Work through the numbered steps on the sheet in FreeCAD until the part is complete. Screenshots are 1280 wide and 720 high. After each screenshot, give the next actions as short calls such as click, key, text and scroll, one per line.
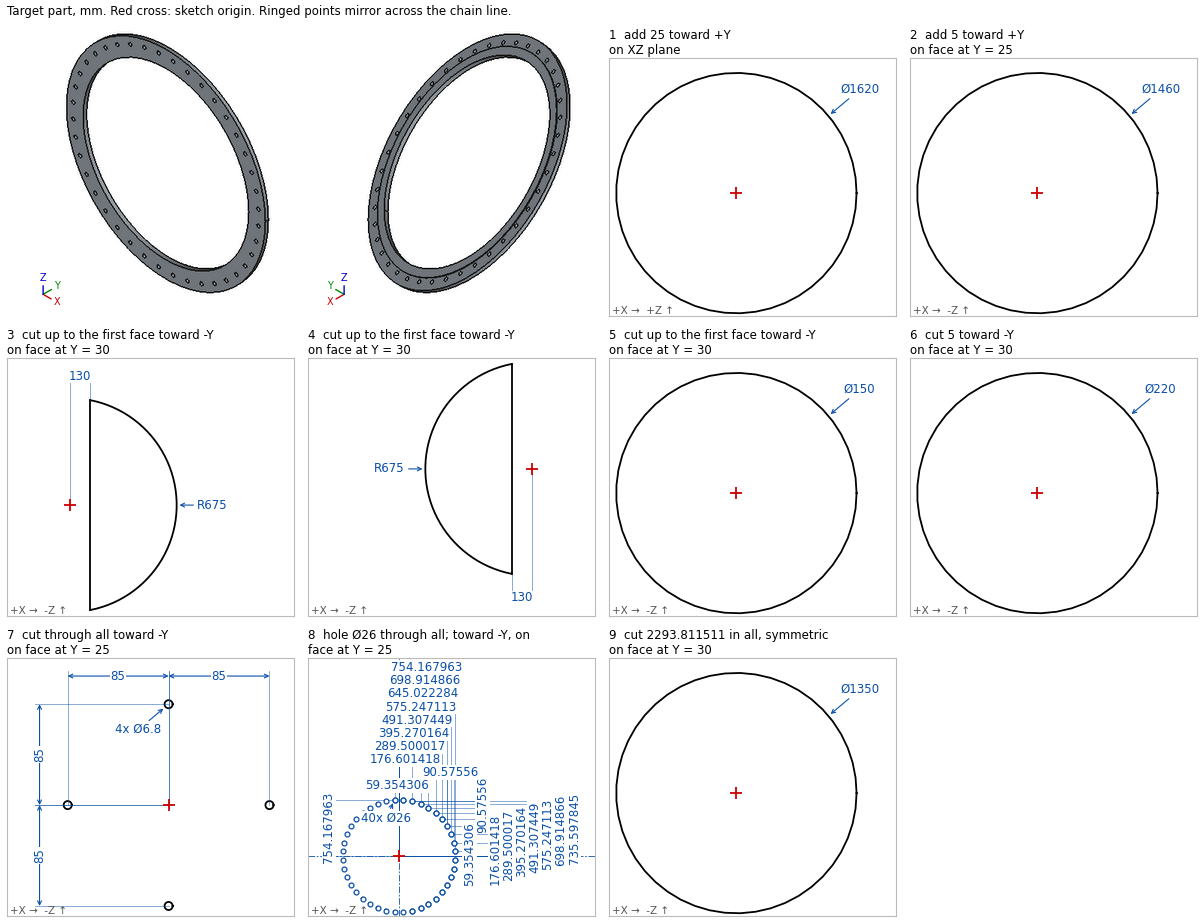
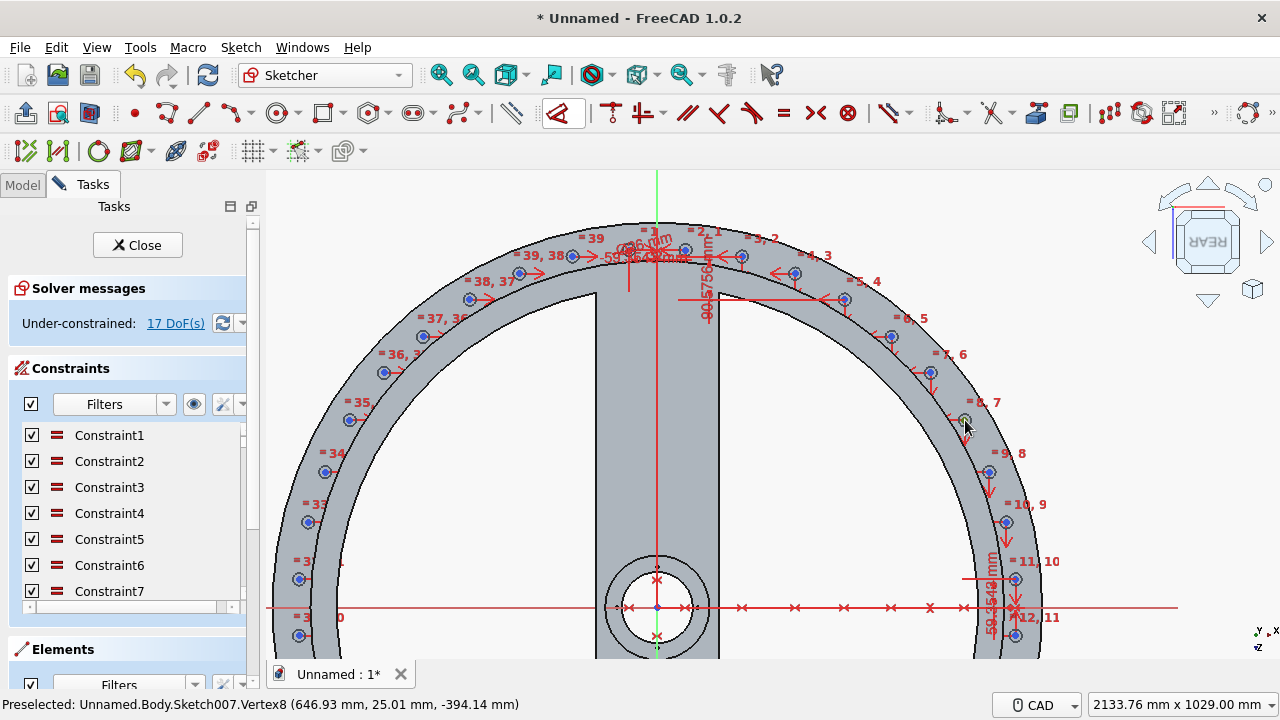
click(1006, 522)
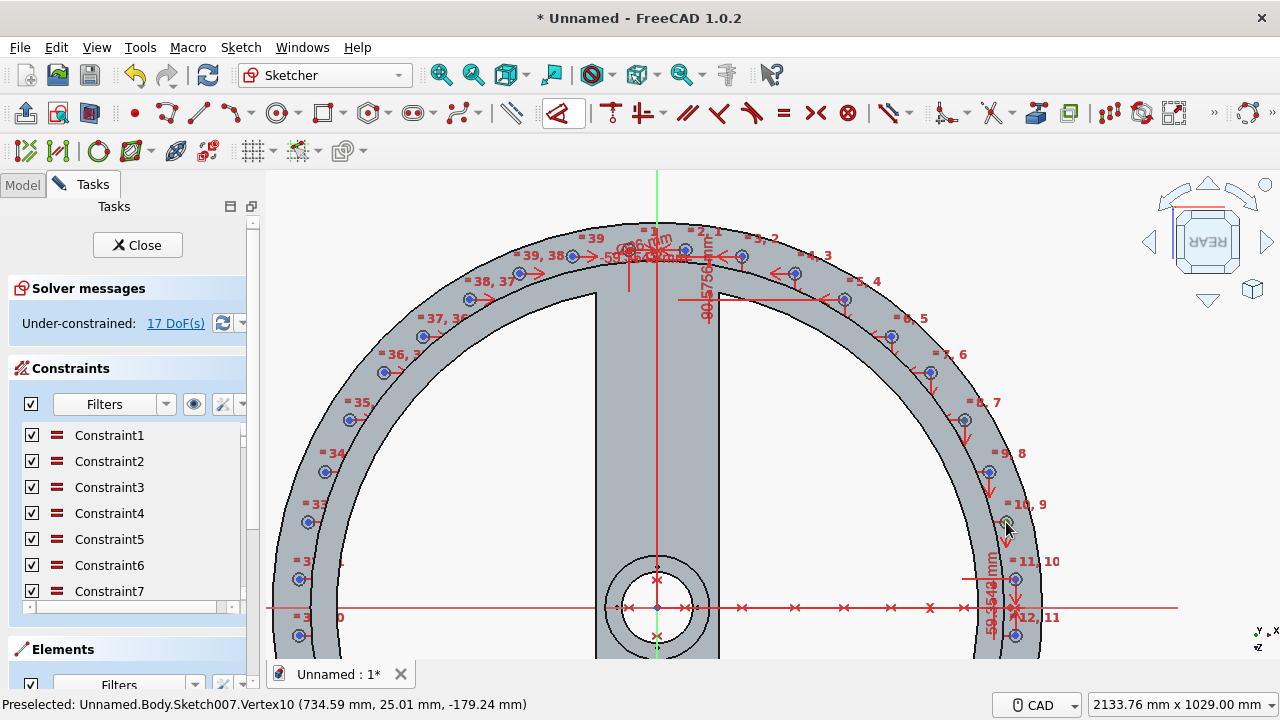
click(580, 114)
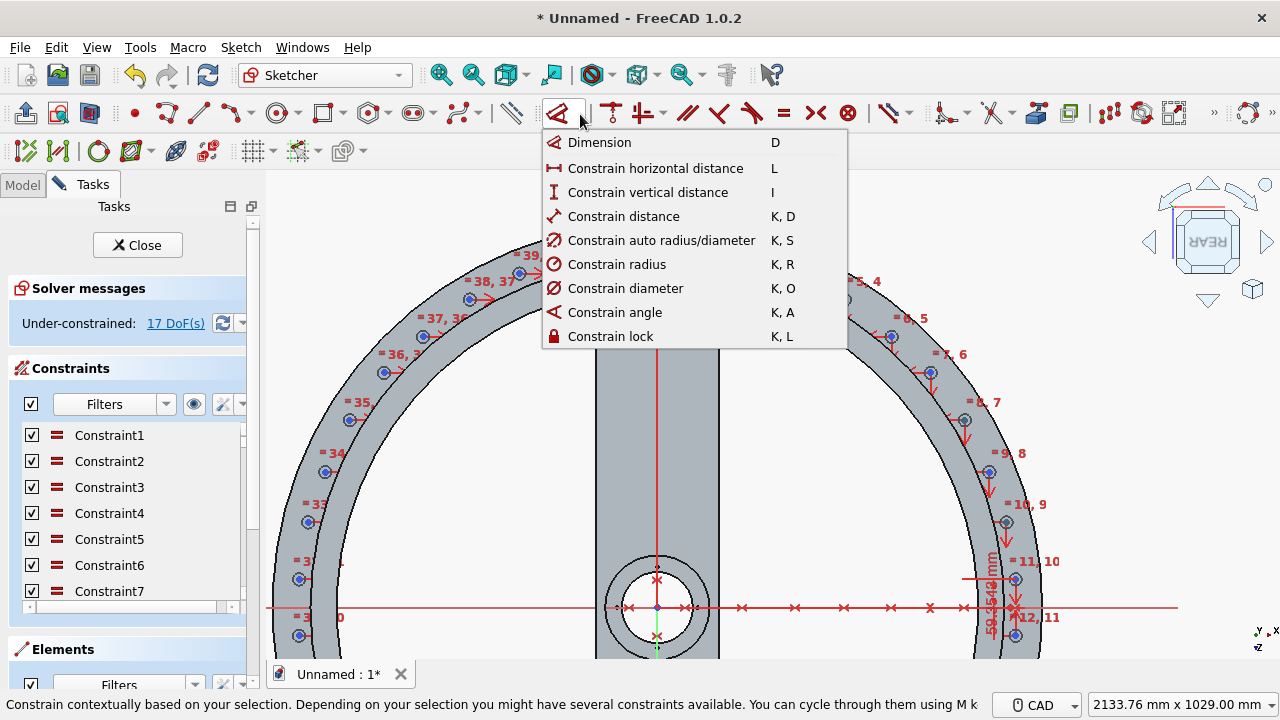
click(695, 168)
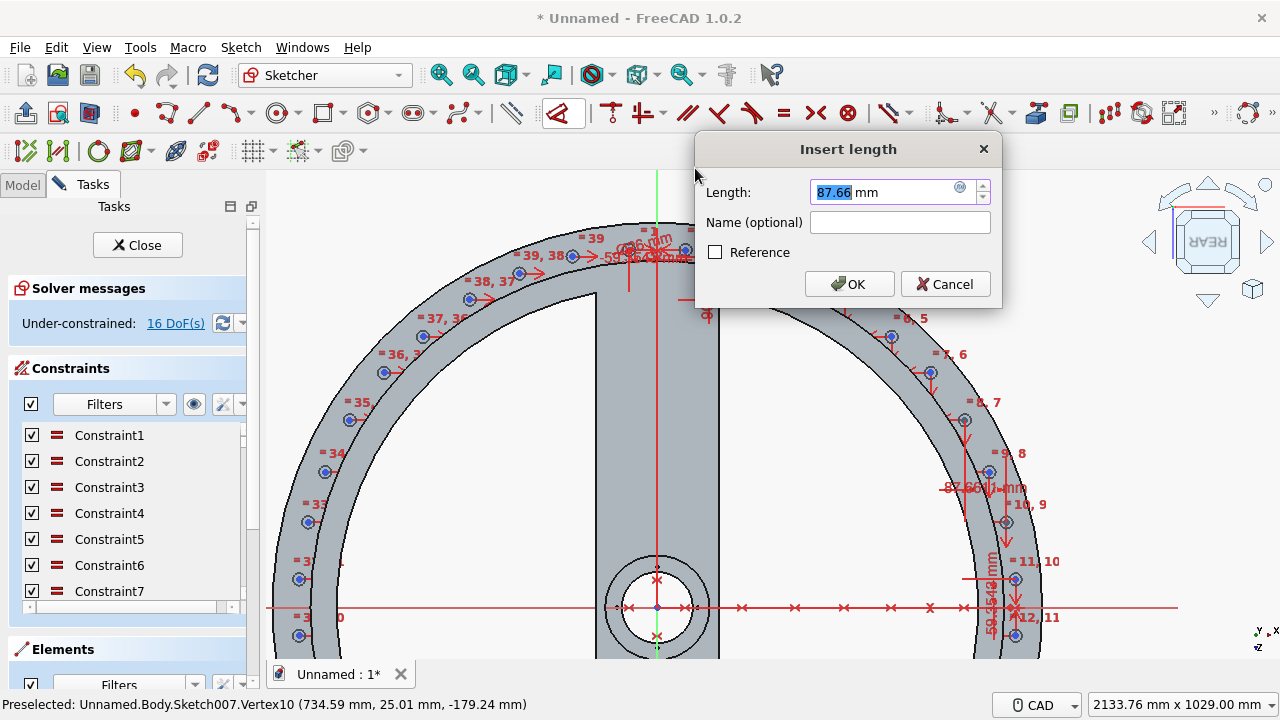
text(90.57556)
key(Return)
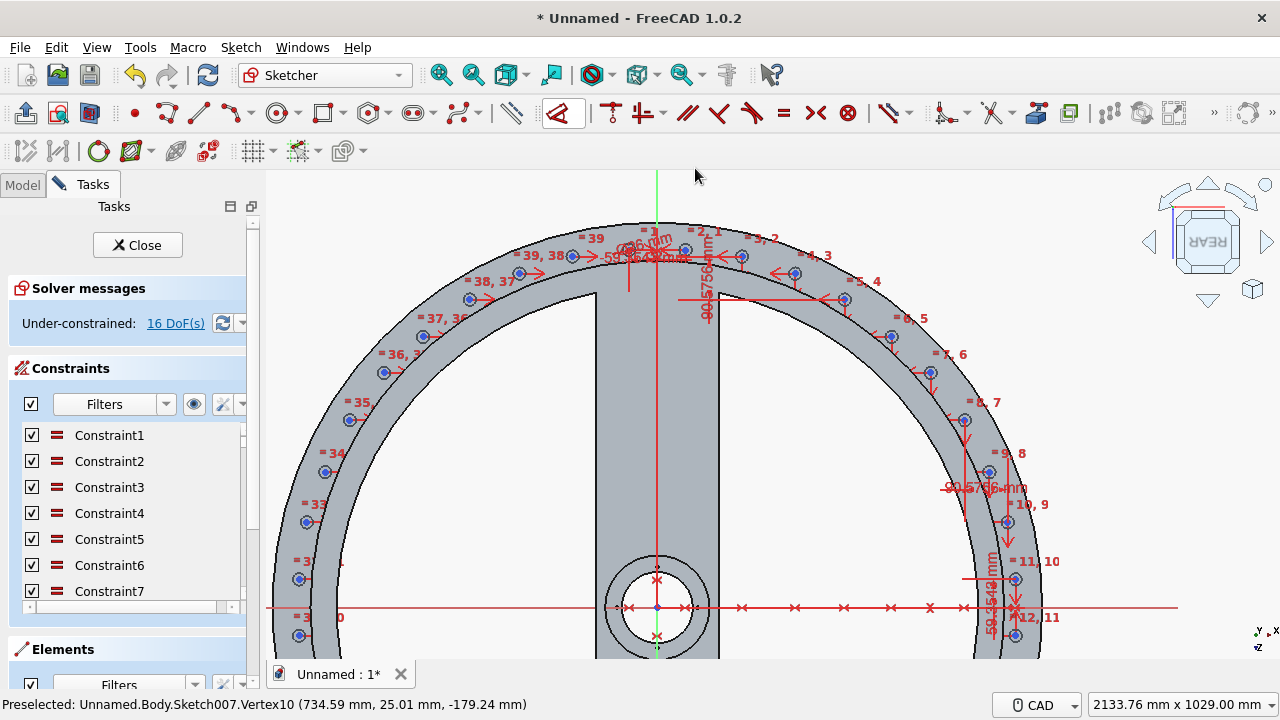
click(629, 250)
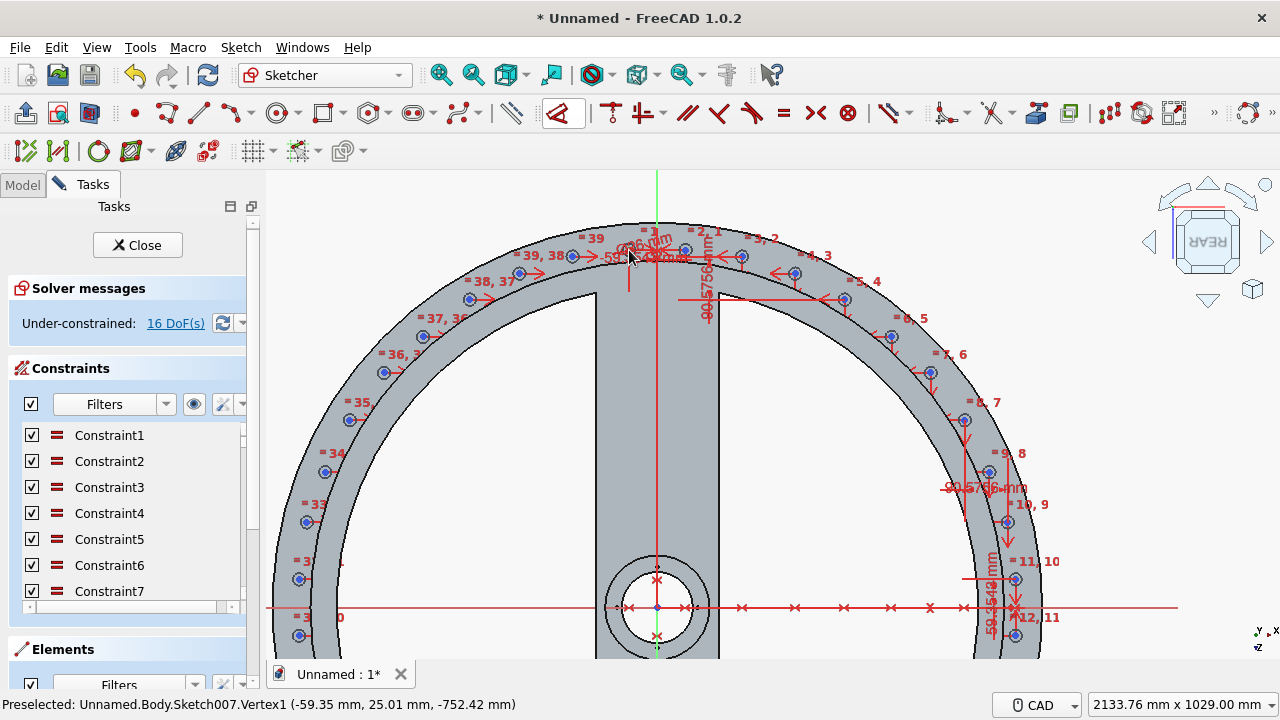
click(580, 114)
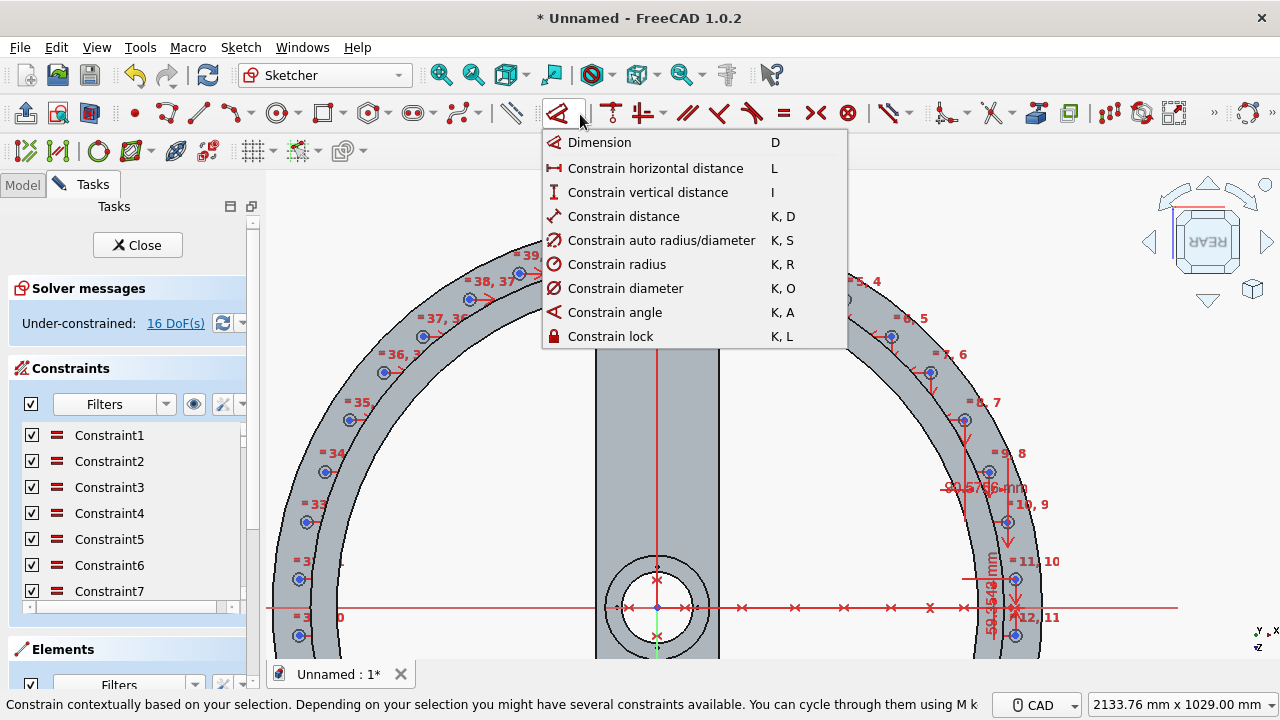
click(695, 192)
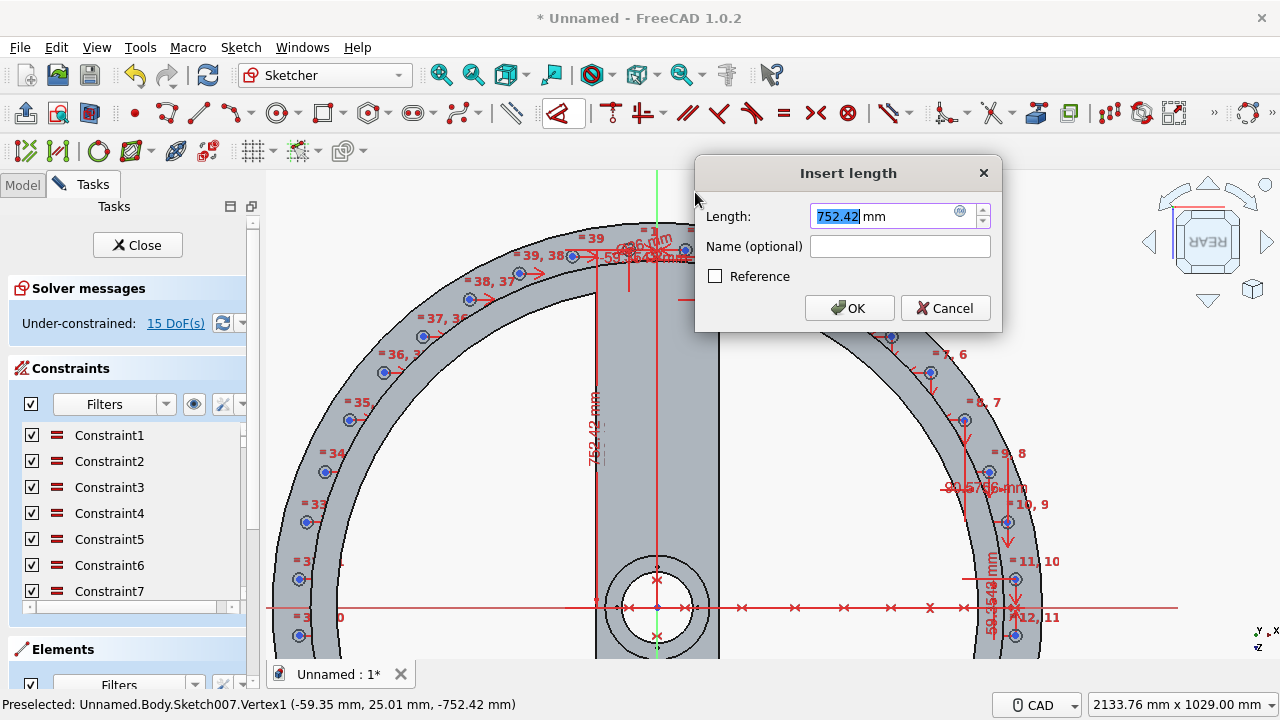
text(754.167963)
key(Return)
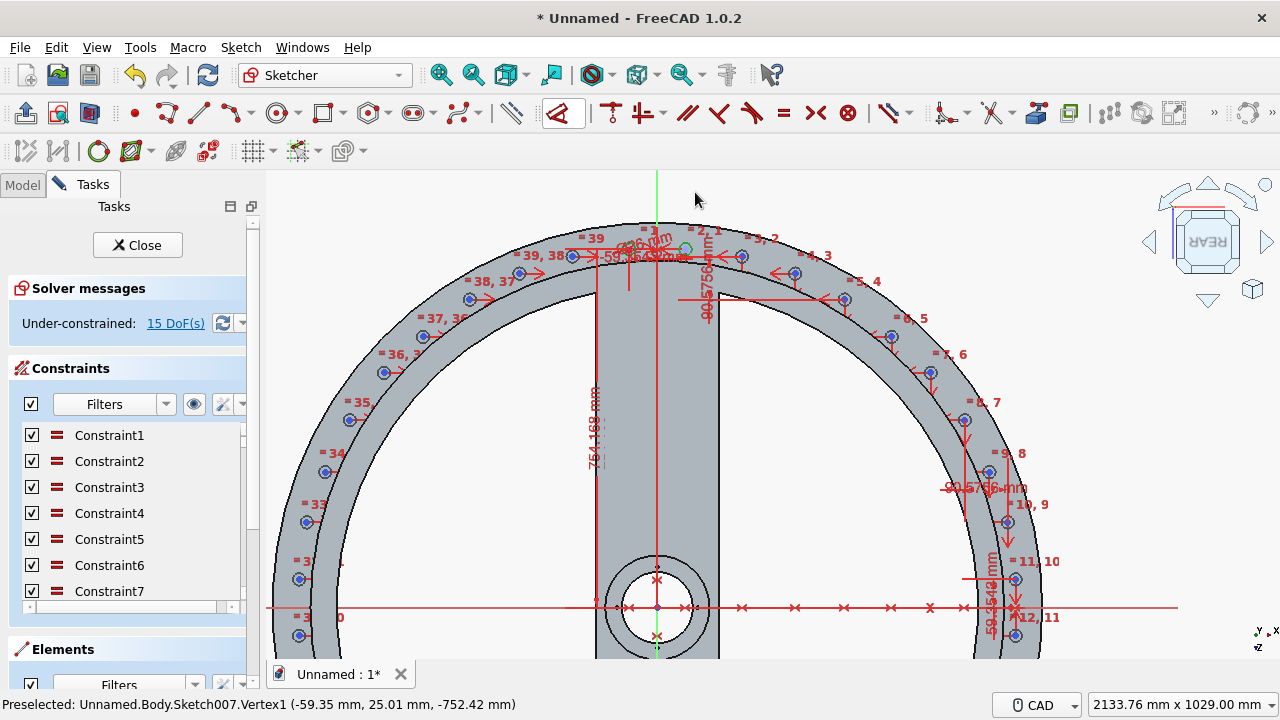
click(742, 257)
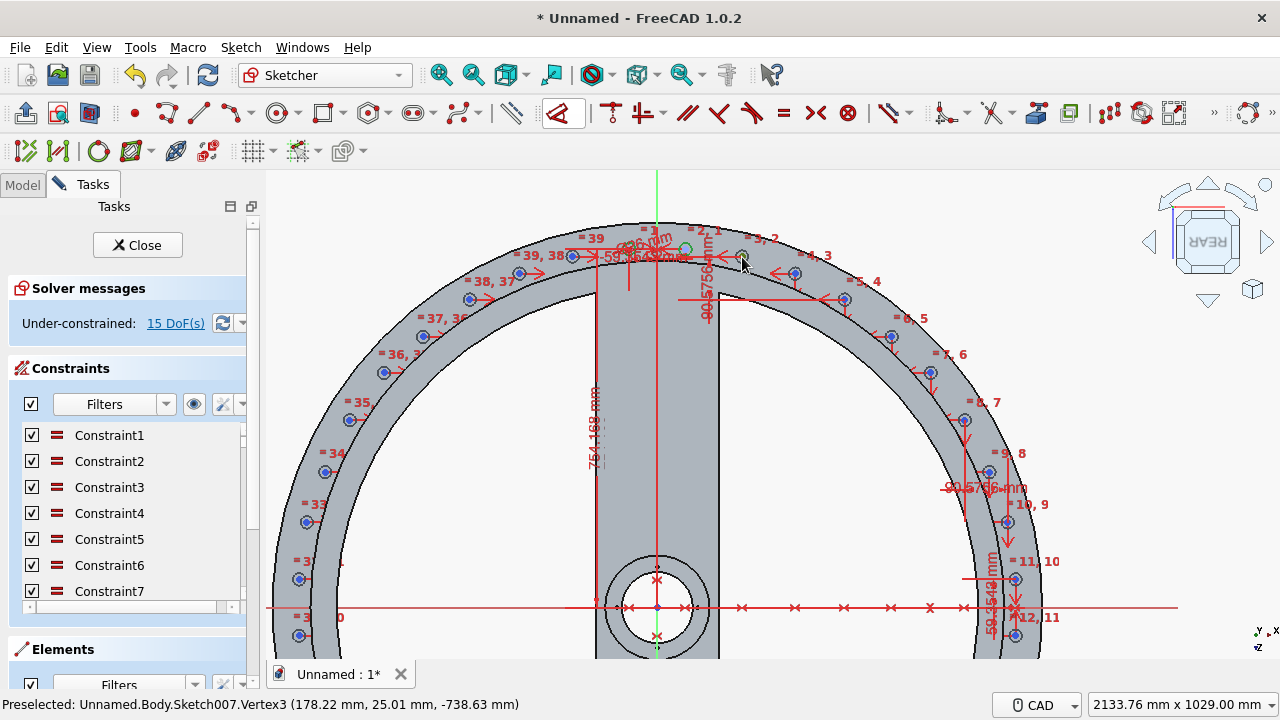
key(l)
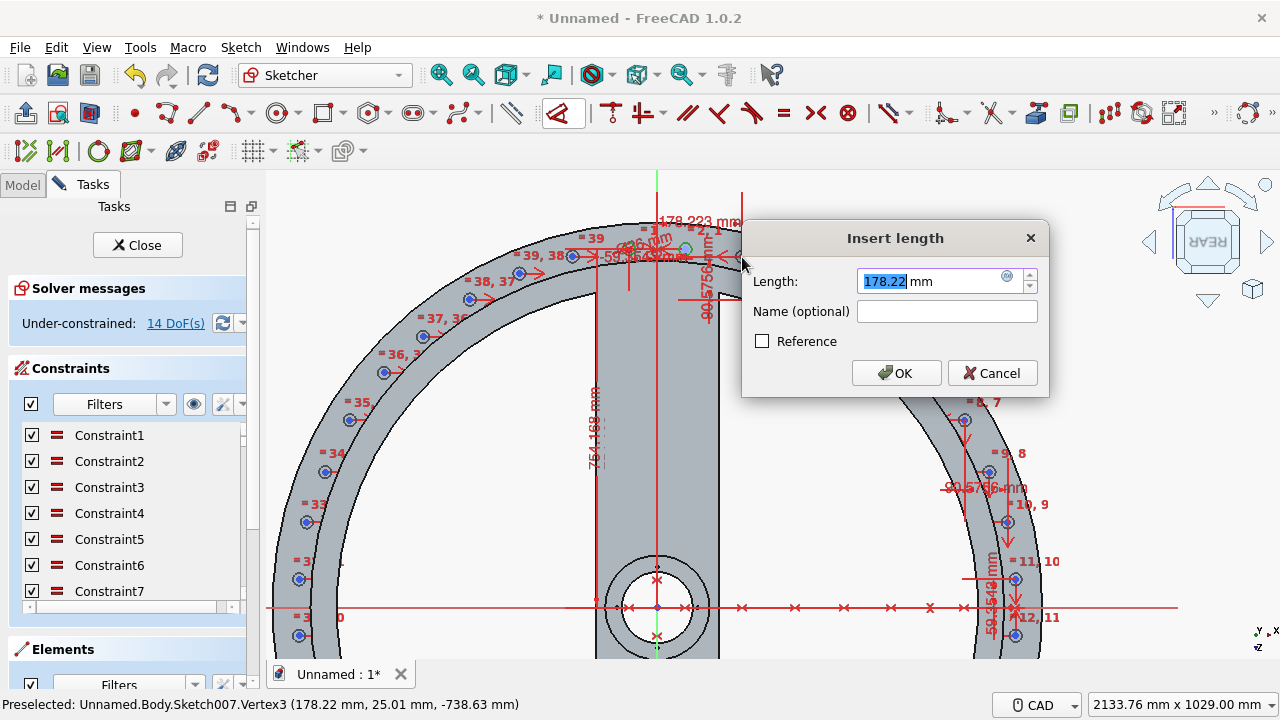
text(176.601418)
key(Return)